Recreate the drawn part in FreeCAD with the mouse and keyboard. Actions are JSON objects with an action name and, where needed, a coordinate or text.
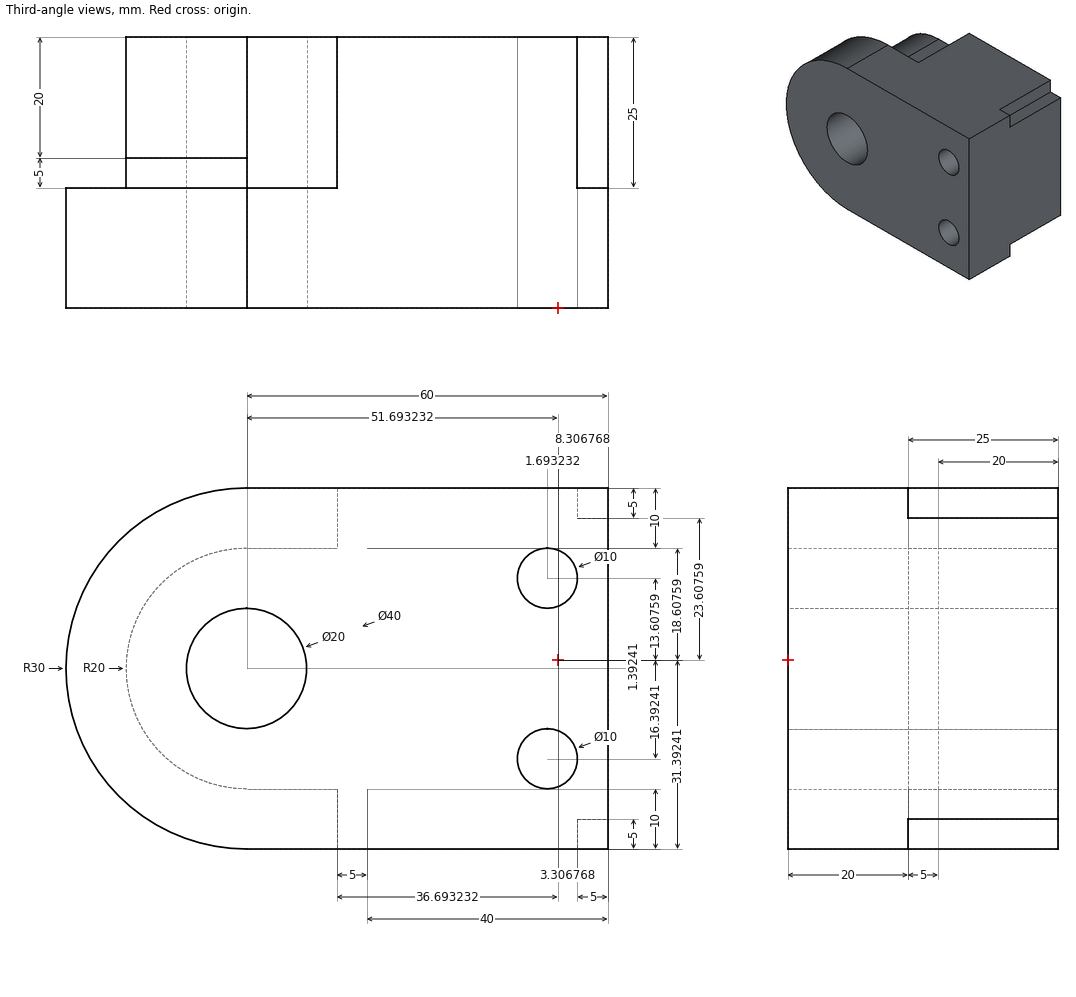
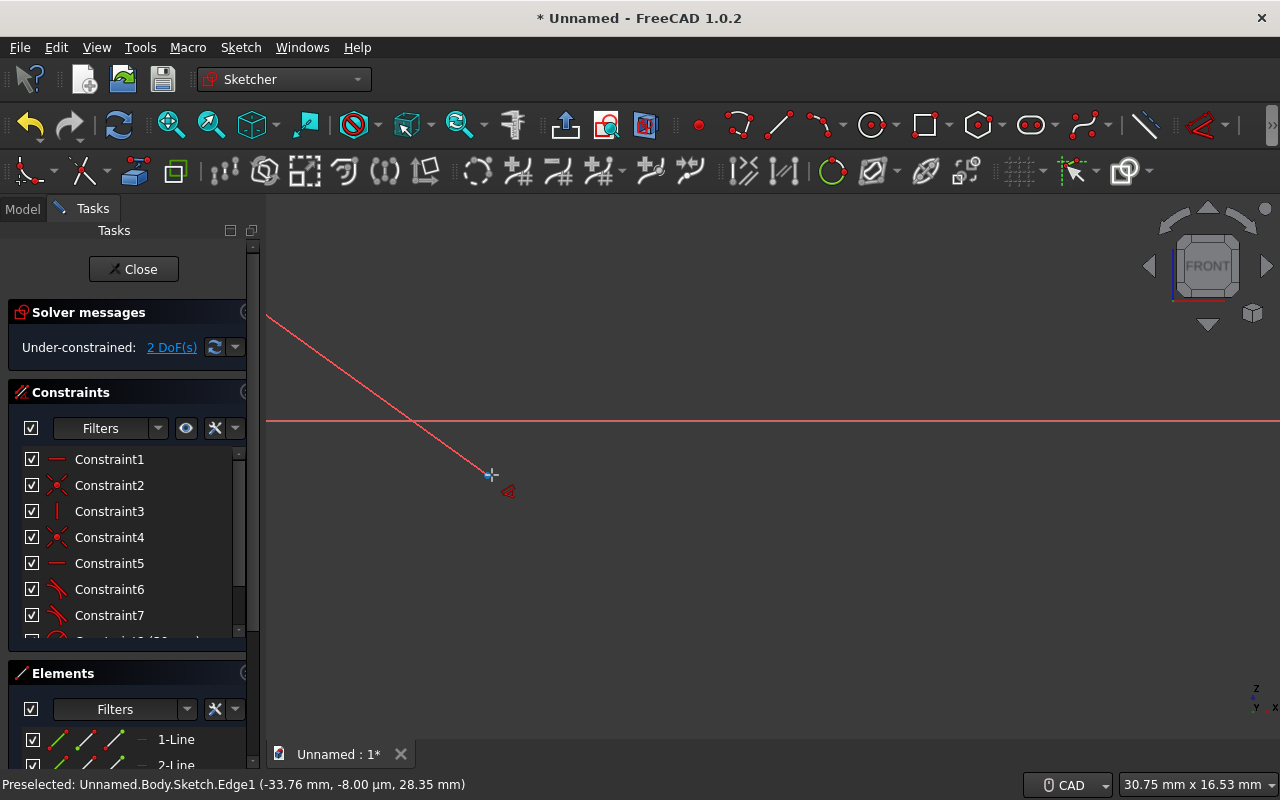
{"action": "left_click", "coordinate": [488, 475]}
{"action": "left_click", "coordinate": [454, 448]}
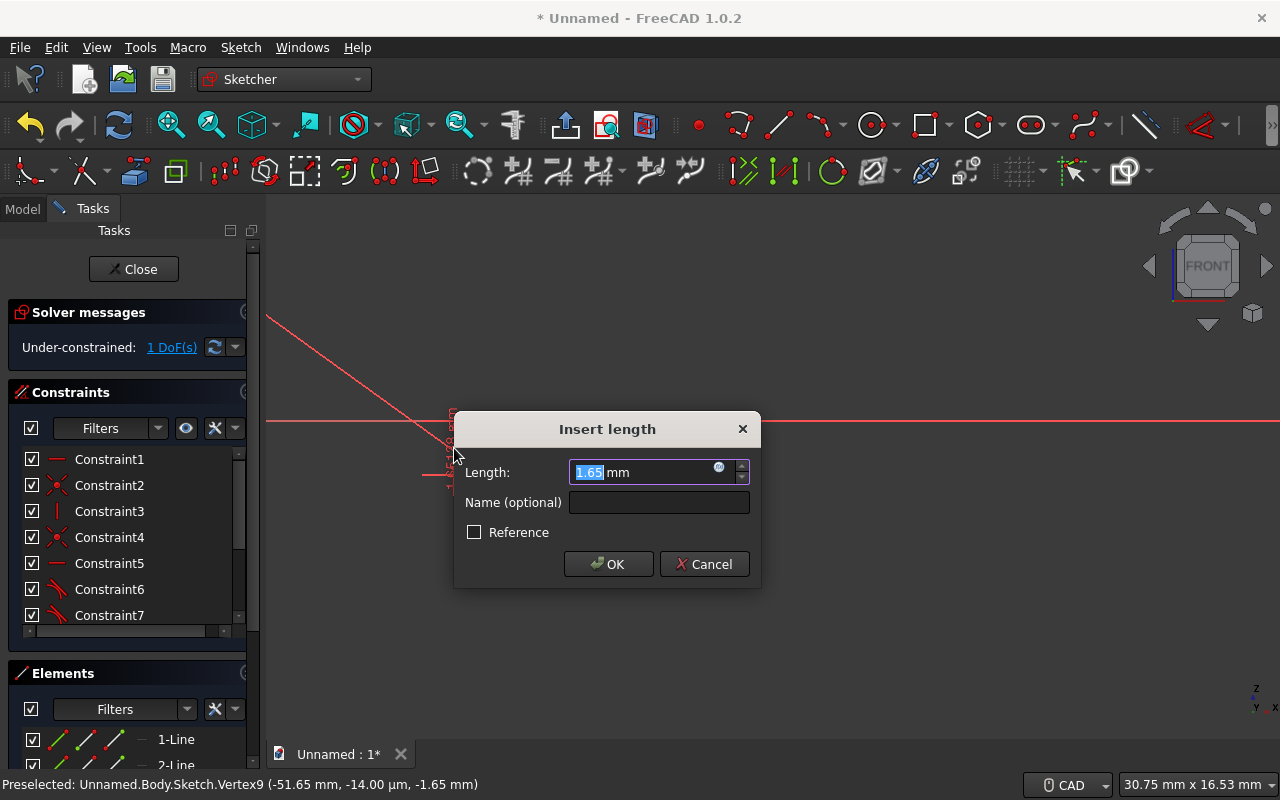
{"action": "type", "text": "1.39241"}
{"action": "key", "text": "Return"}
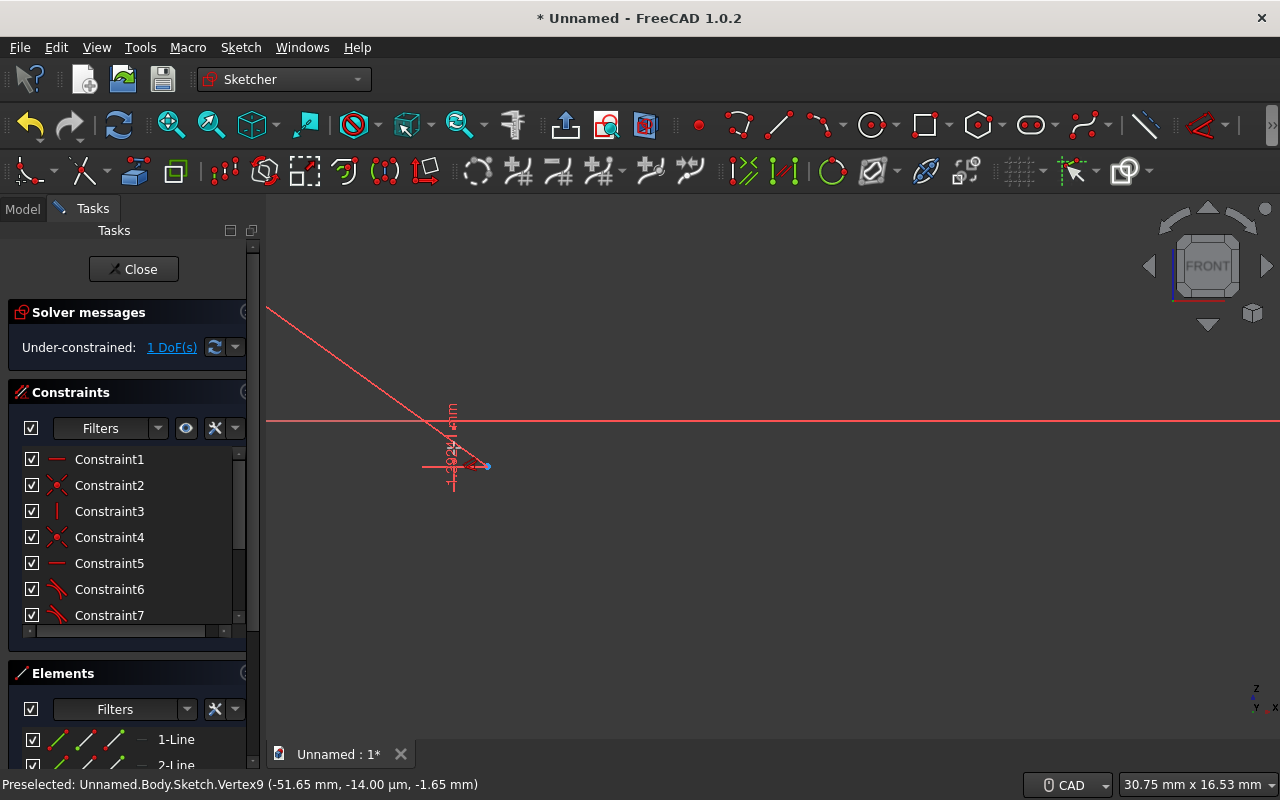
{"action": "scroll", "coordinate": [650, 466], "scroll_direction": "down", "scroll_amount": 9}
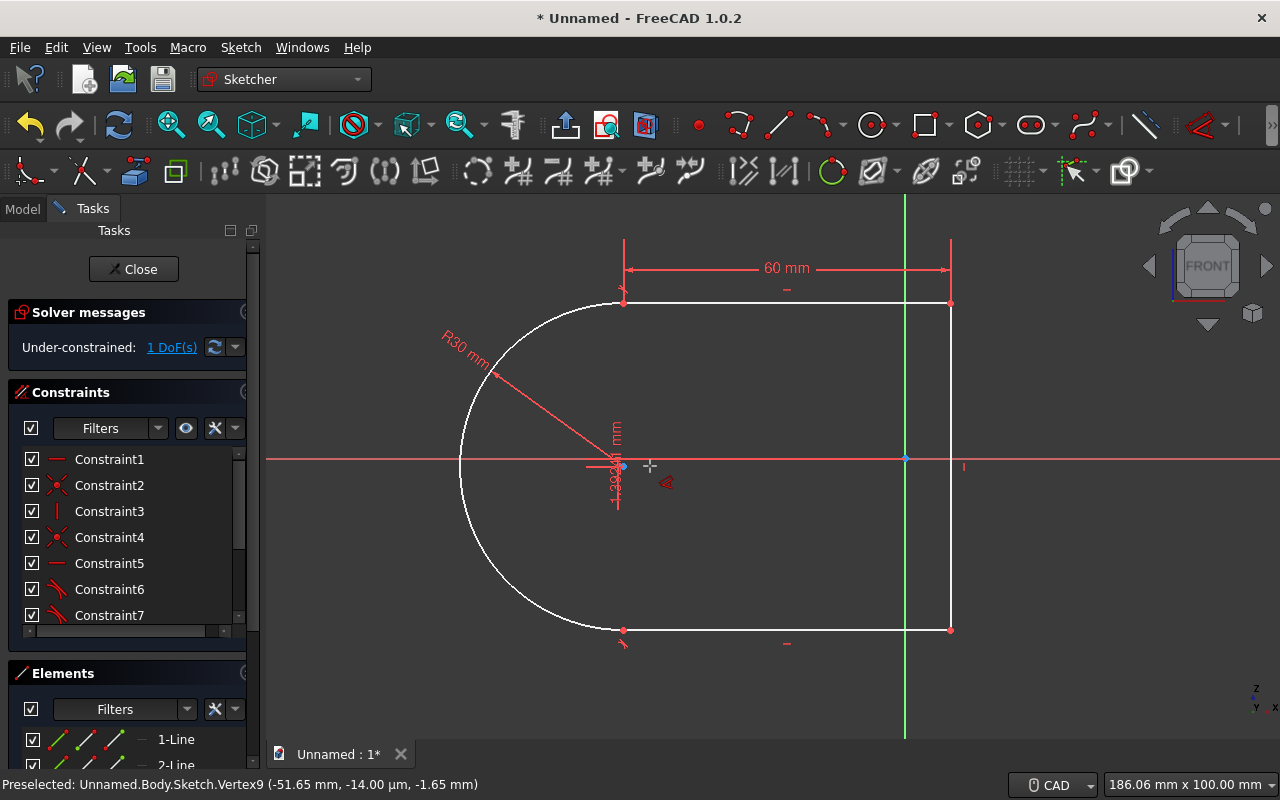
{"action": "left_click", "coordinate": [951, 303]}
{"action": "left_click", "coordinate": [928, 269]}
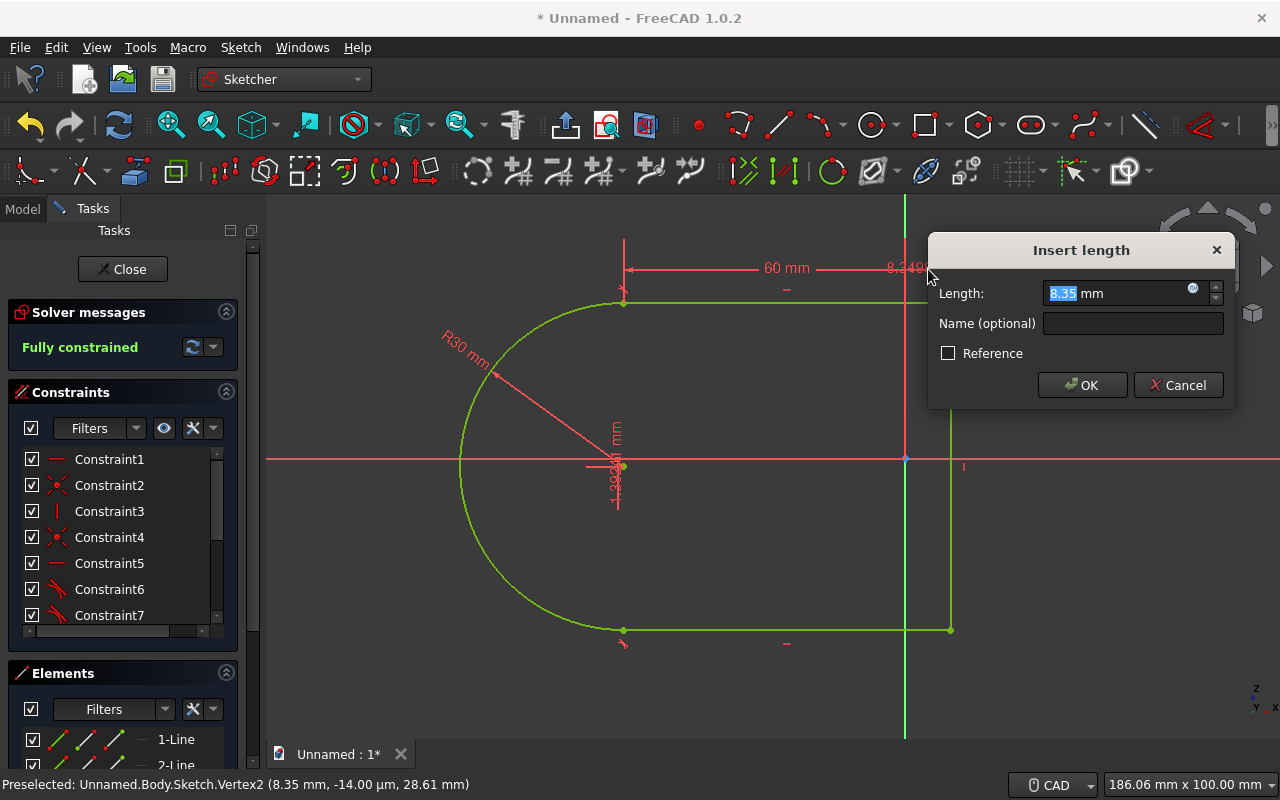
{"action": "type", "text": "8.306768"}
{"action": "key", "text": "Return"}
{"action": "key", "text": "Escape"}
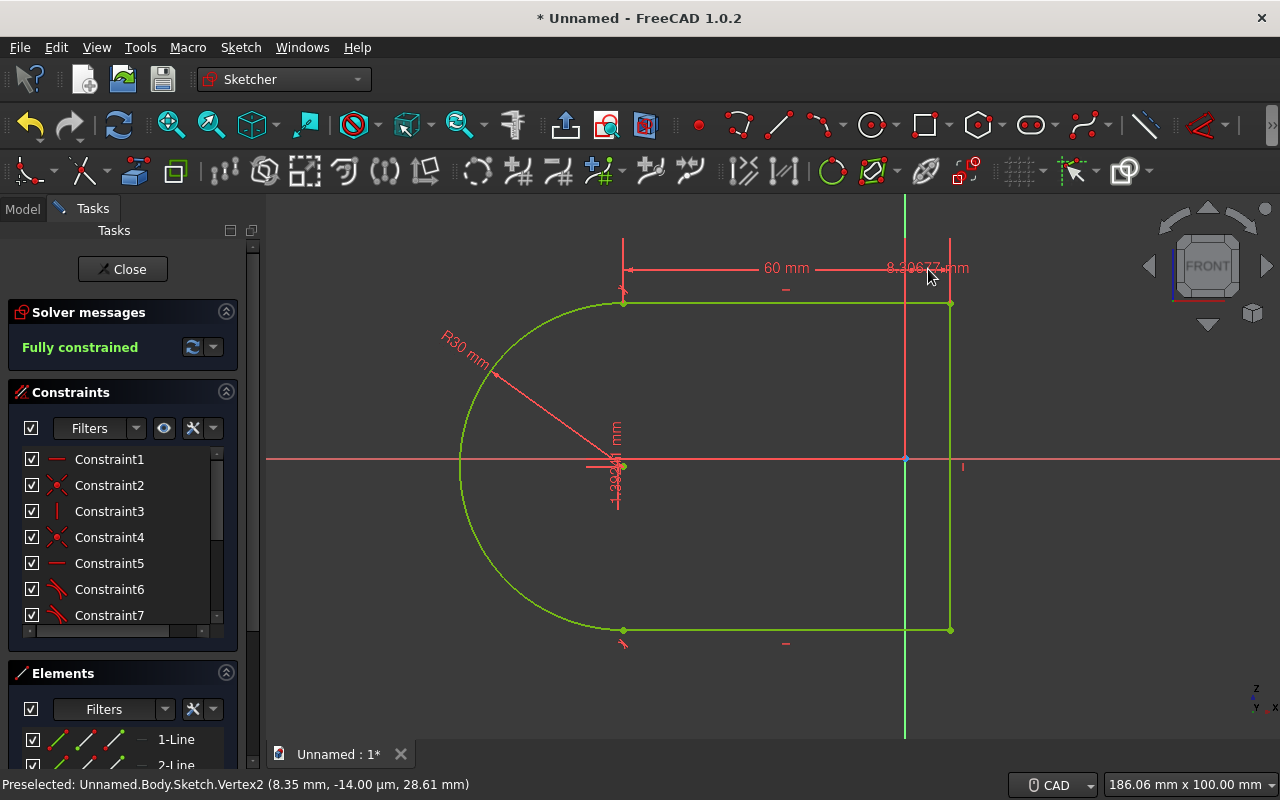
{"action": "left_click", "coordinate": [123, 269]}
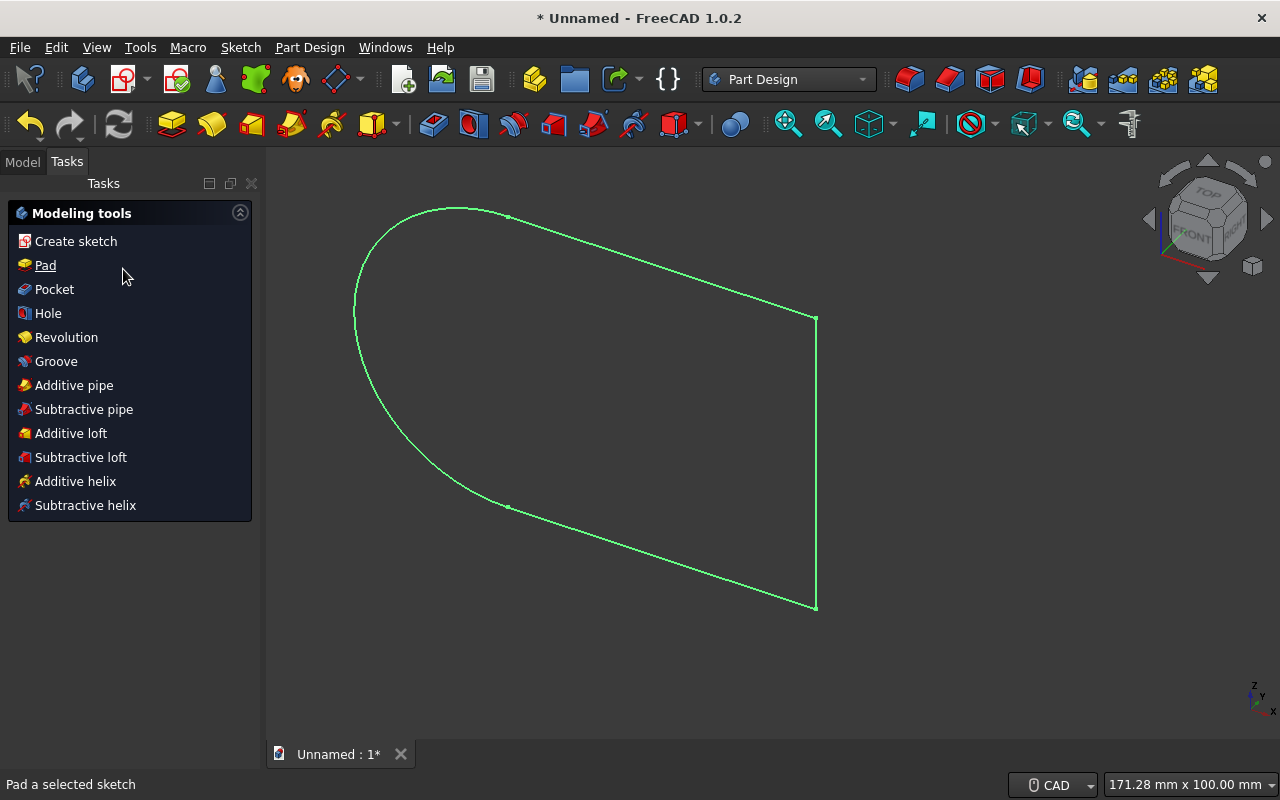
{"action": "left_click", "coordinate": [172, 124]}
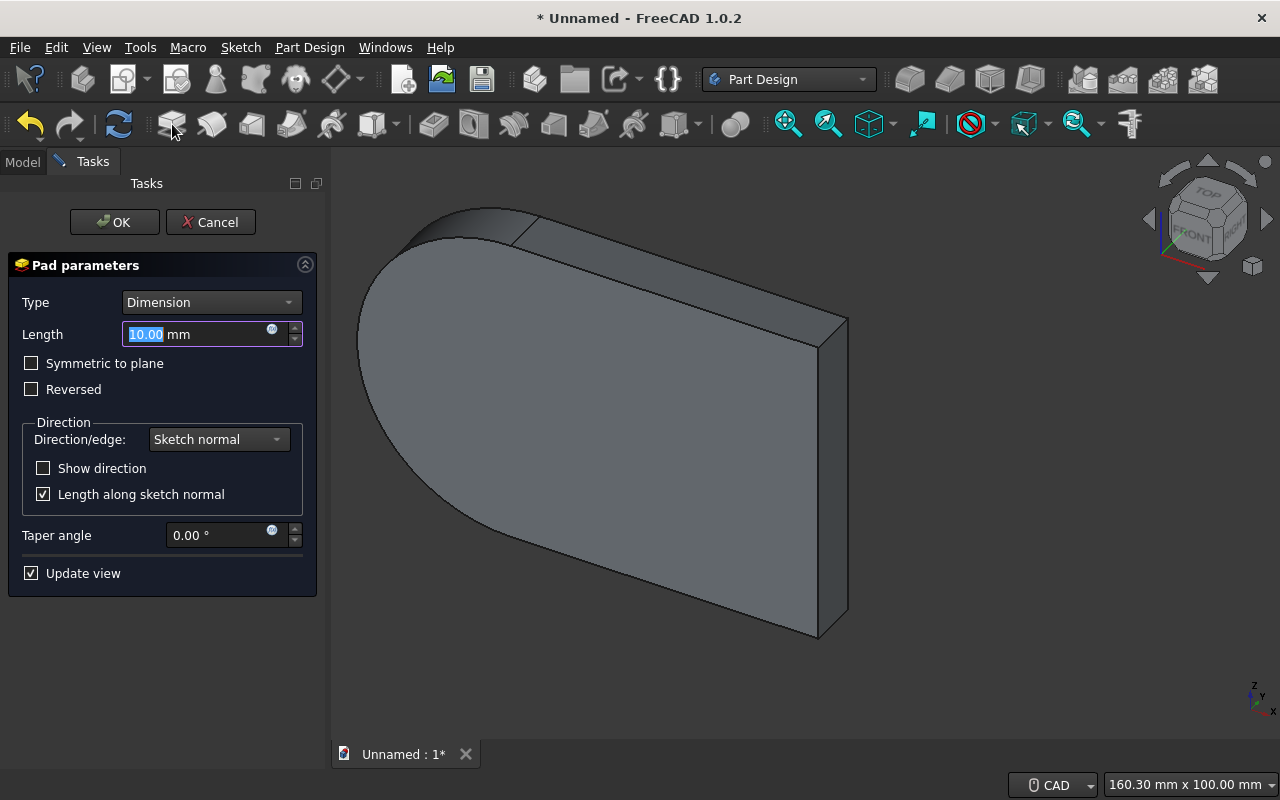
{"action": "type", "text": "20"}
{"action": "key", "text": "Tab"}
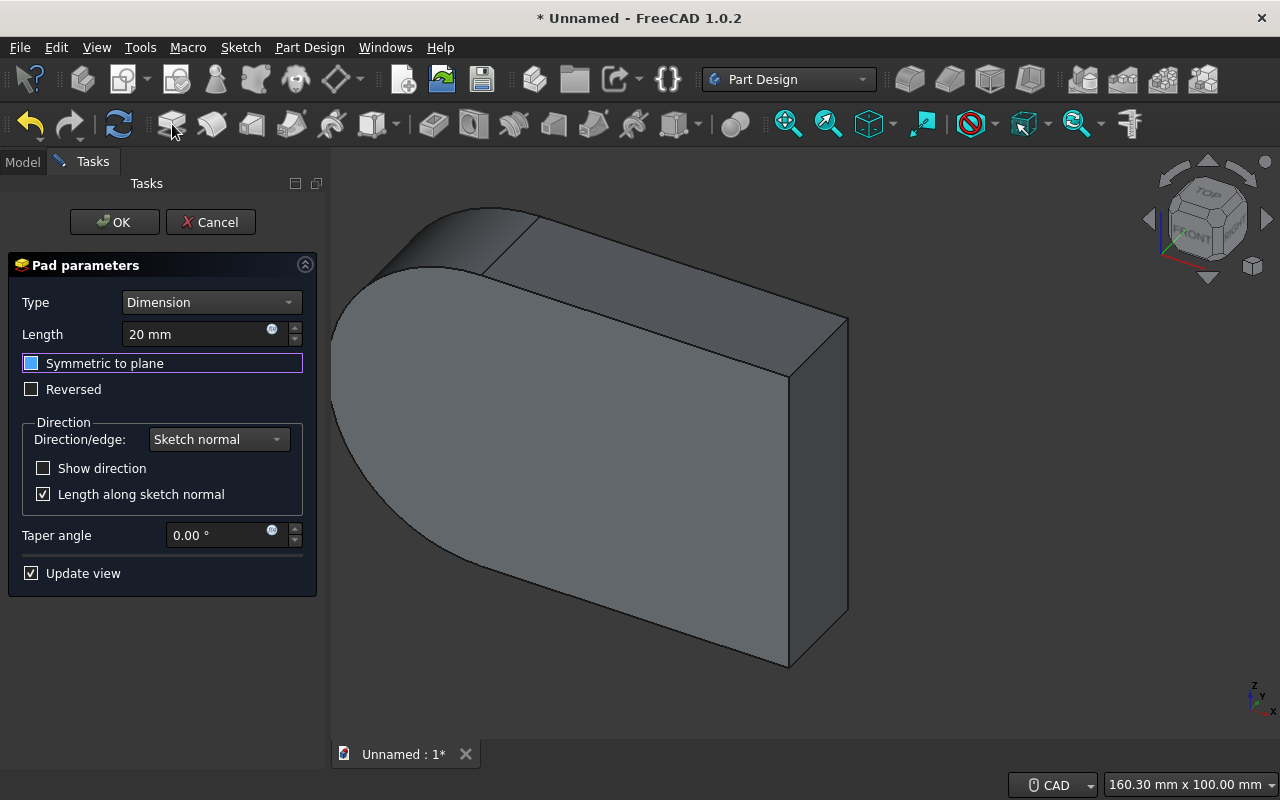
{"action": "left_click", "coordinate": [30, 389]}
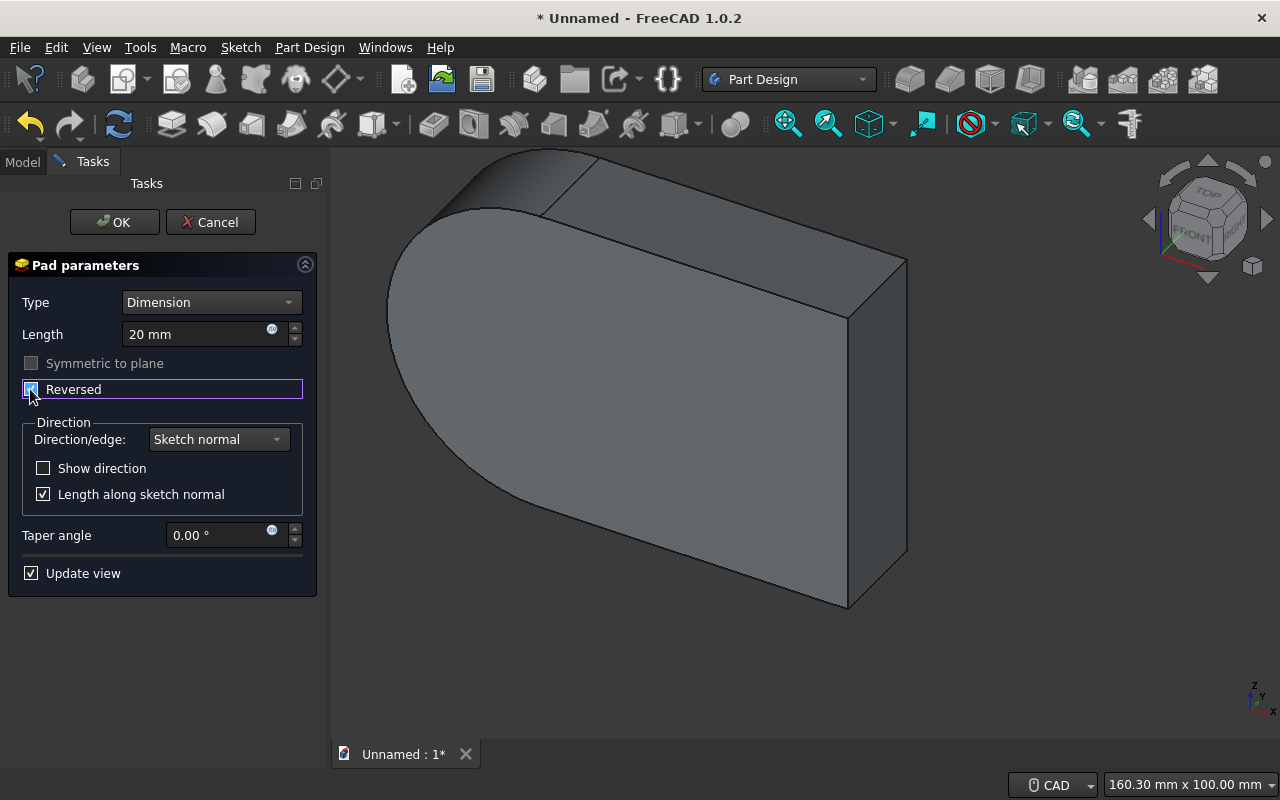
{"action": "left_click", "coordinate": [115, 222]}